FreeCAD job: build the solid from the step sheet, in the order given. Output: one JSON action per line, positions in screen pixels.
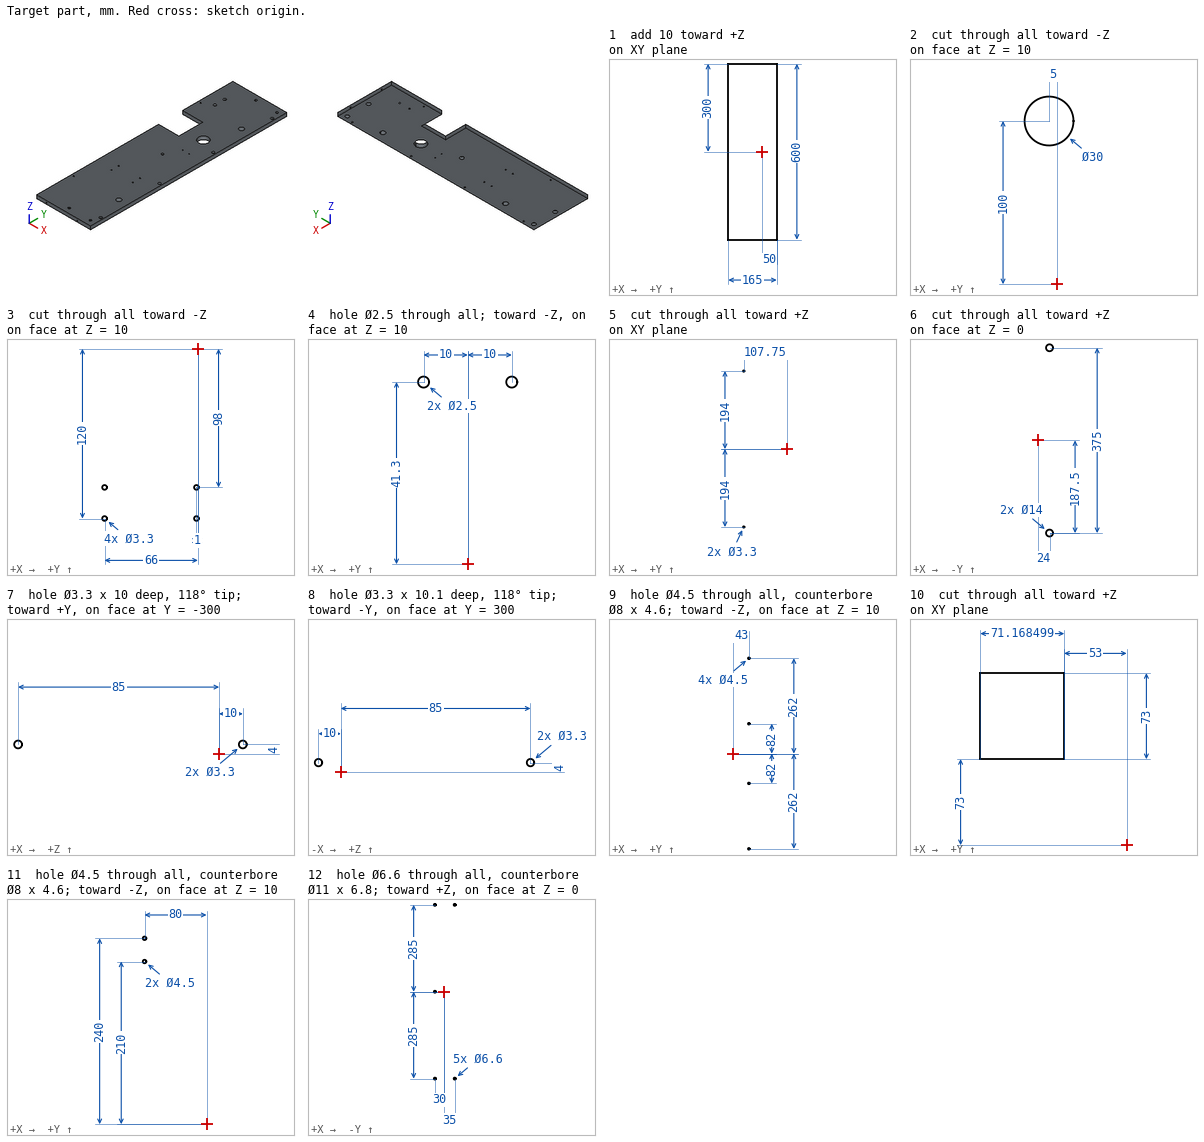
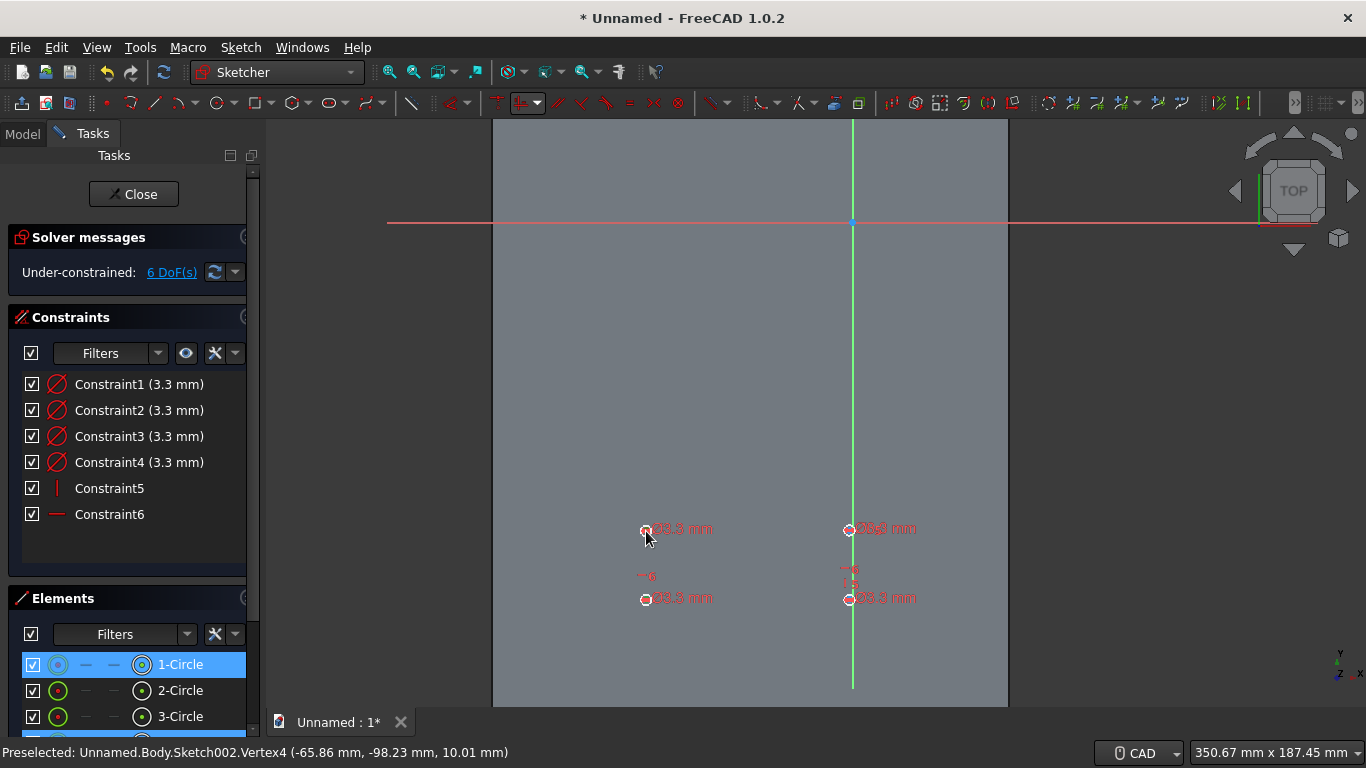
{"action": "left_click", "coordinate": [540, 104]}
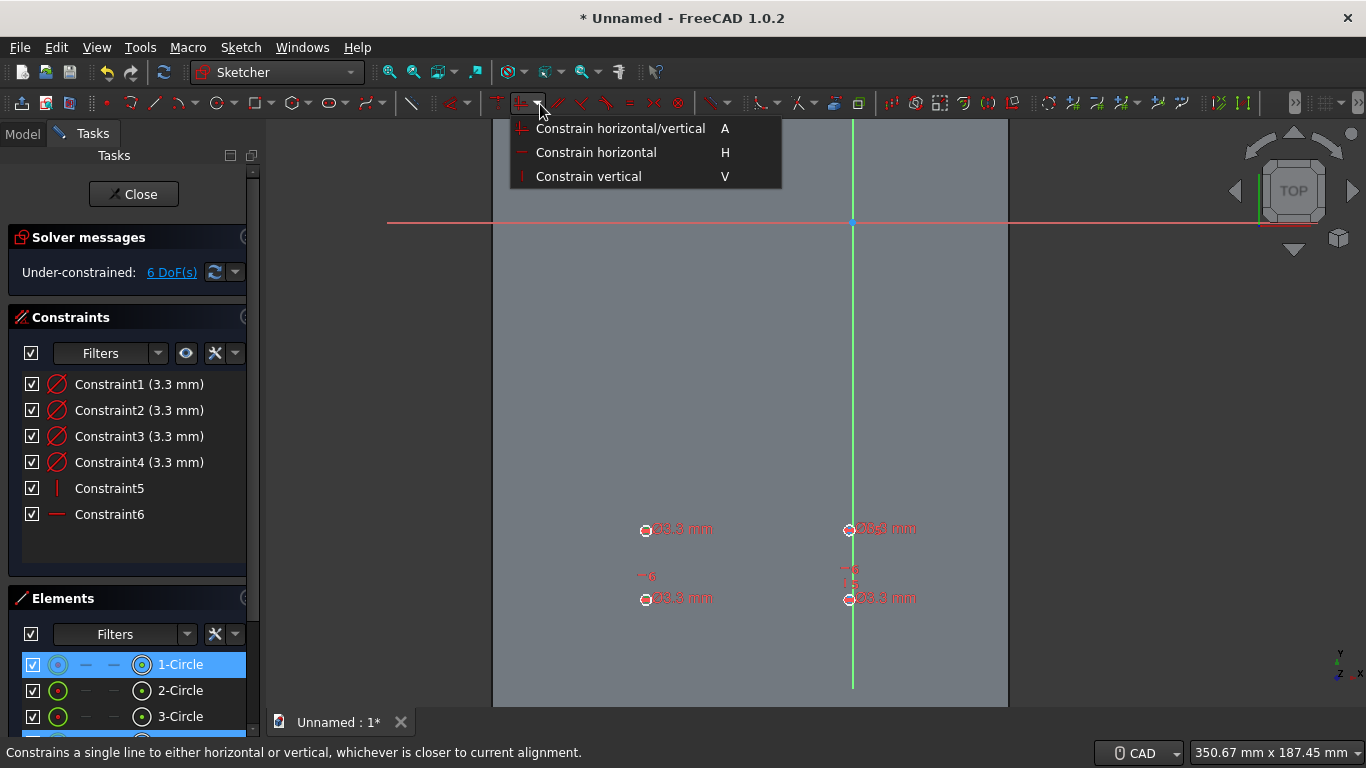
{"action": "left_click", "coordinate": [646, 176]}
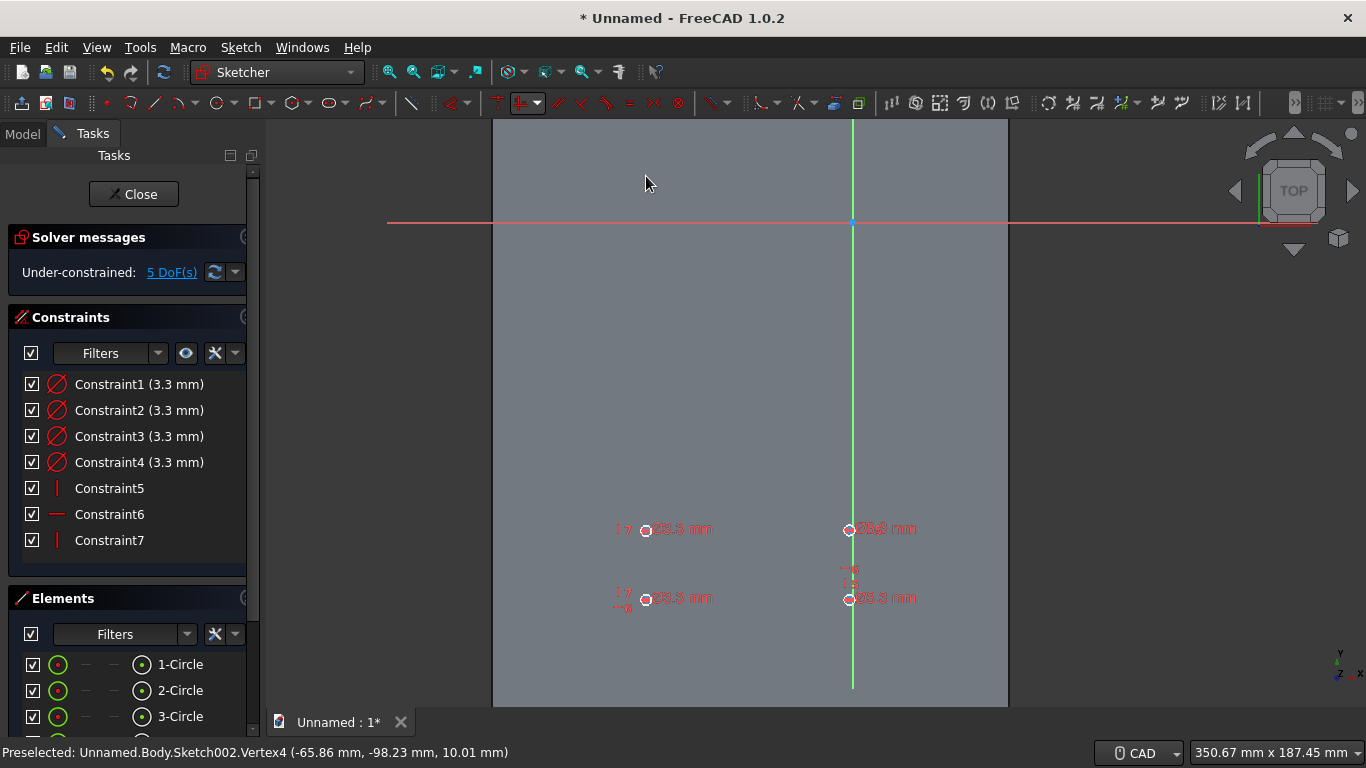
{"action": "left_click", "coordinate": [849, 530]}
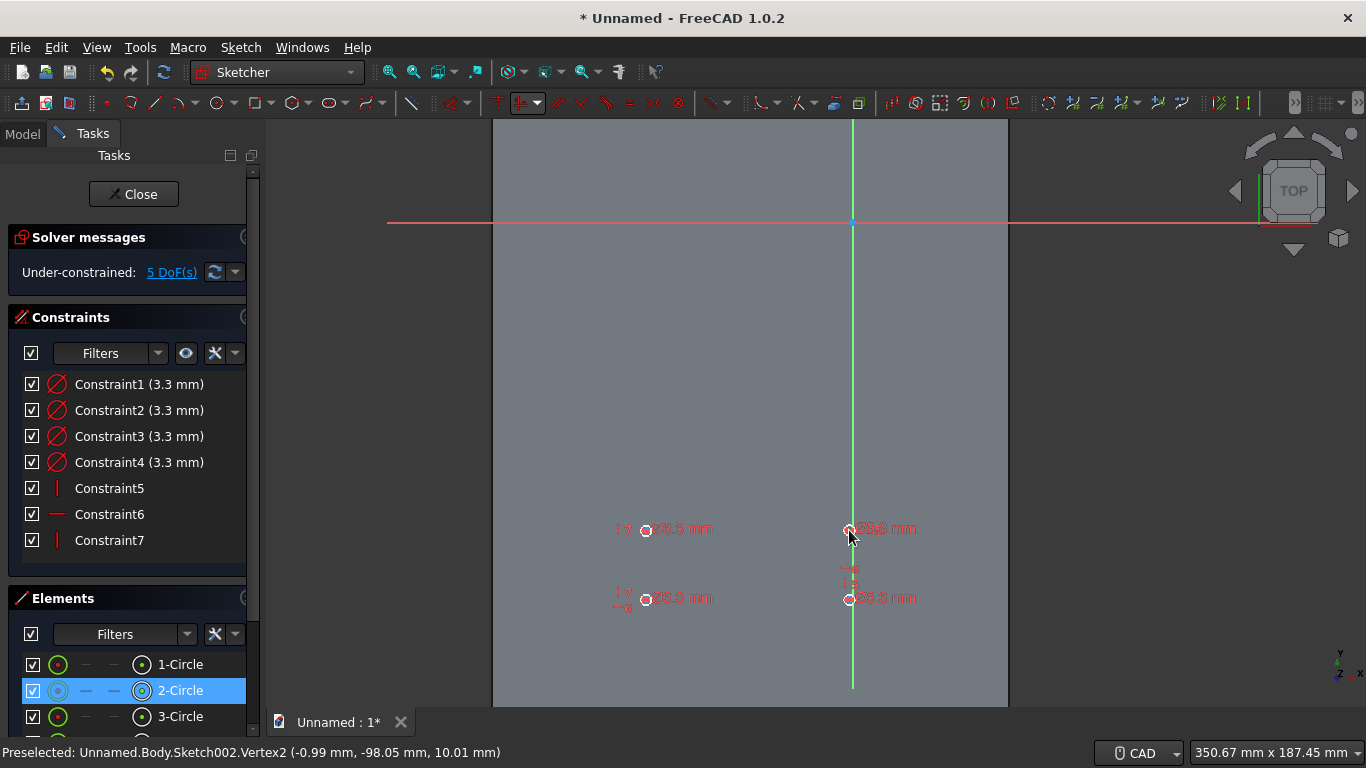
{"action": "left_click", "coordinate": [646, 531]}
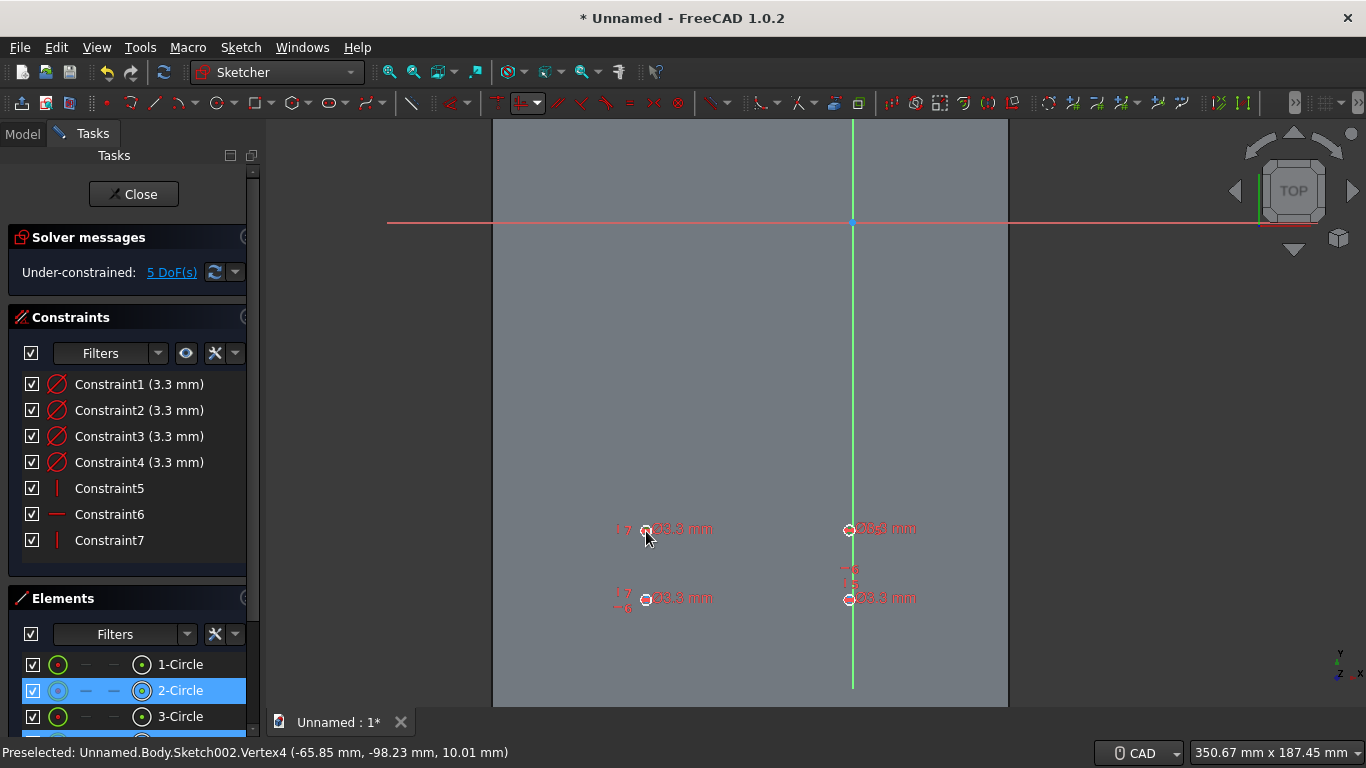
{"action": "left_click", "coordinate": [540, 104]}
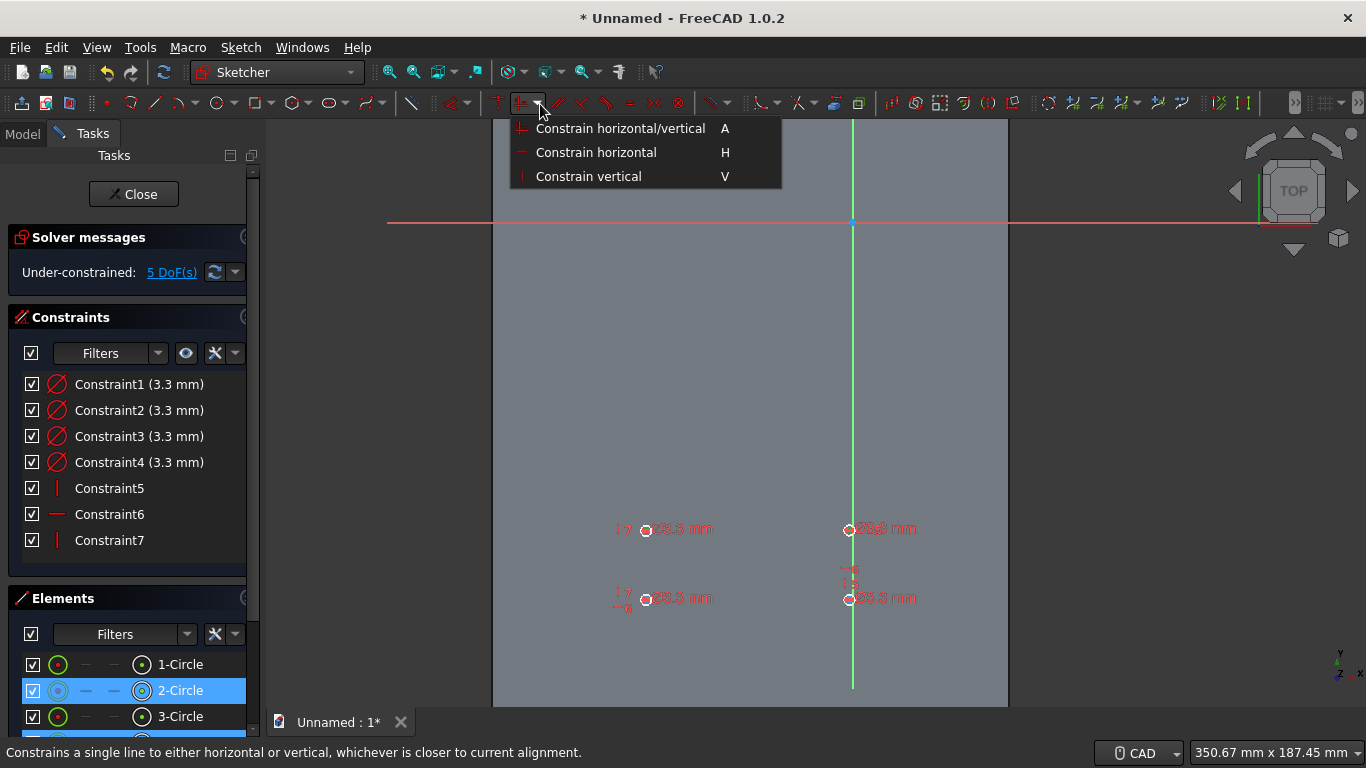
{"action": "left_click", "coordinate": [646, 152]}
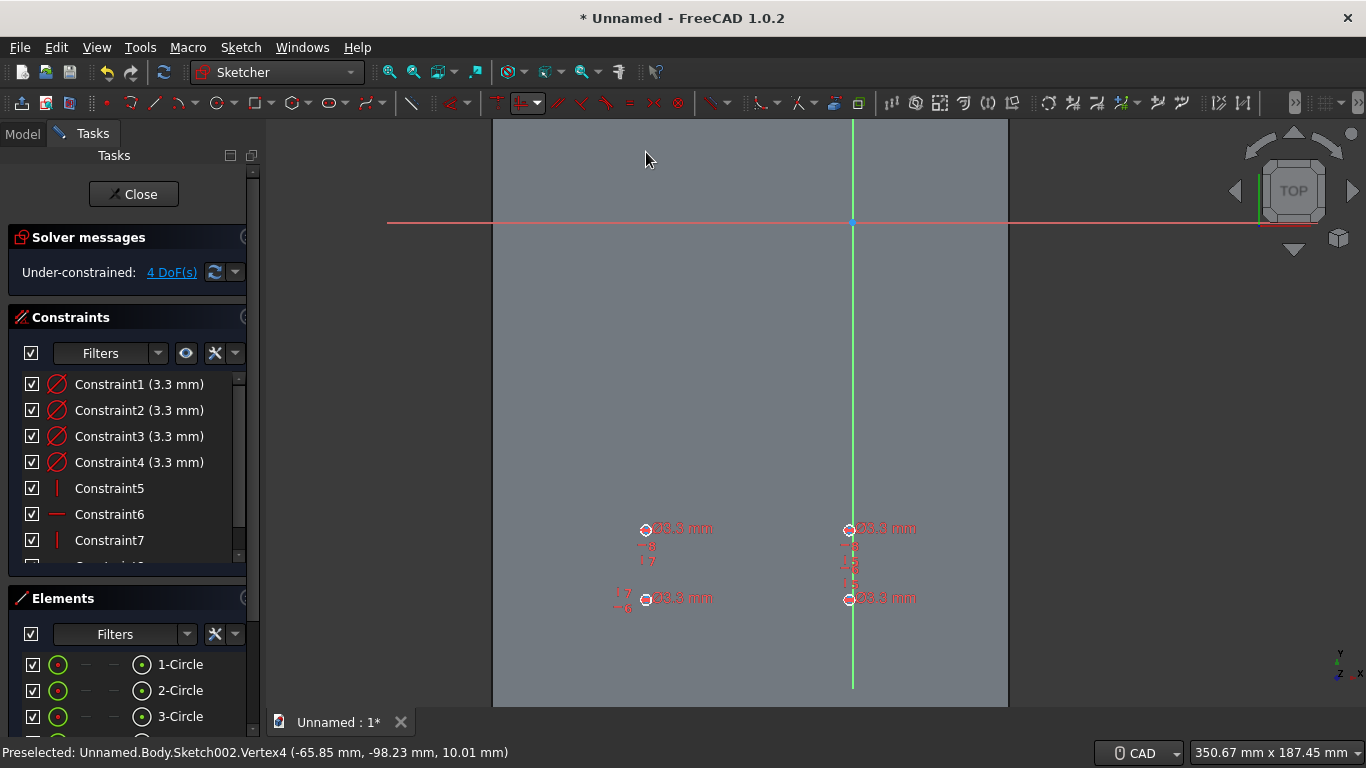
{"action": "left_click", "coordinate": [450, 104]}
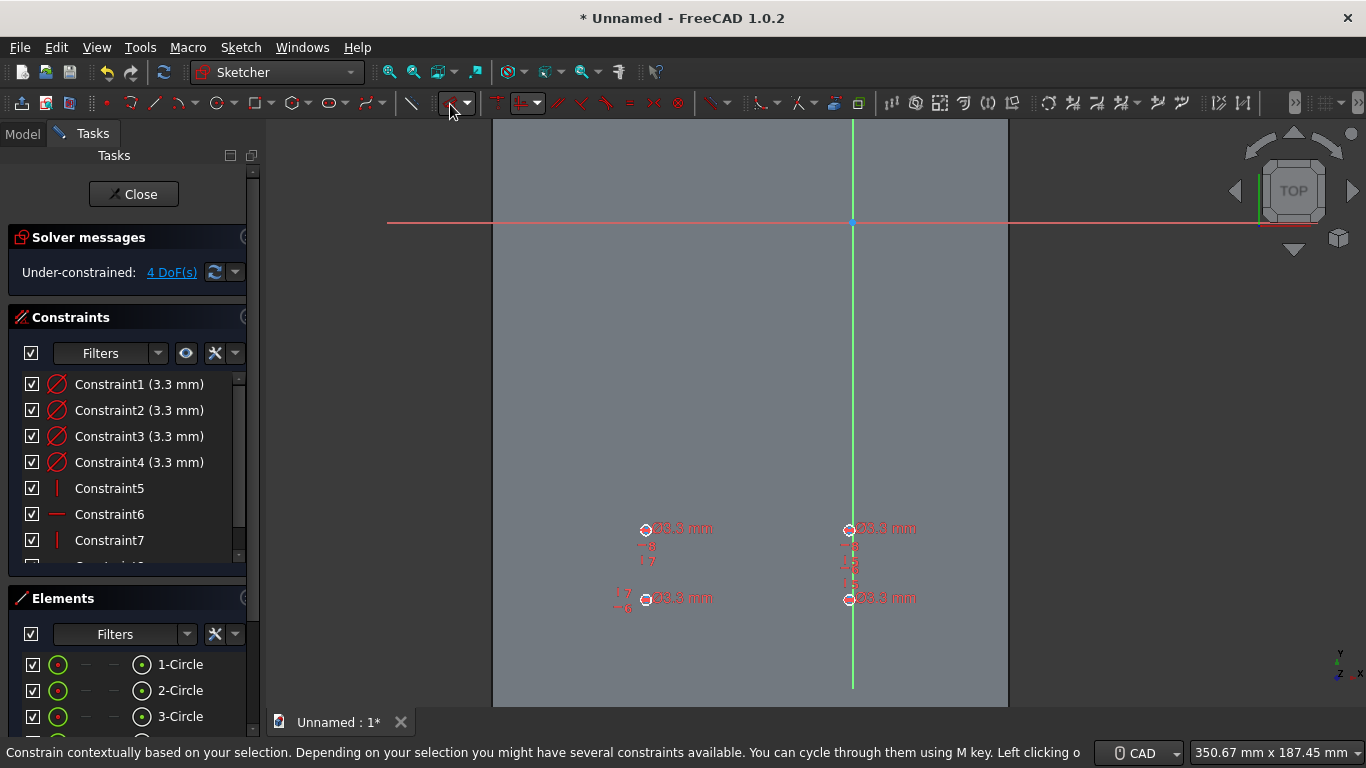
{"action": "scroll", "coordinate": [849, 530], "scroll_direction": "up", "scroll_amount": 13}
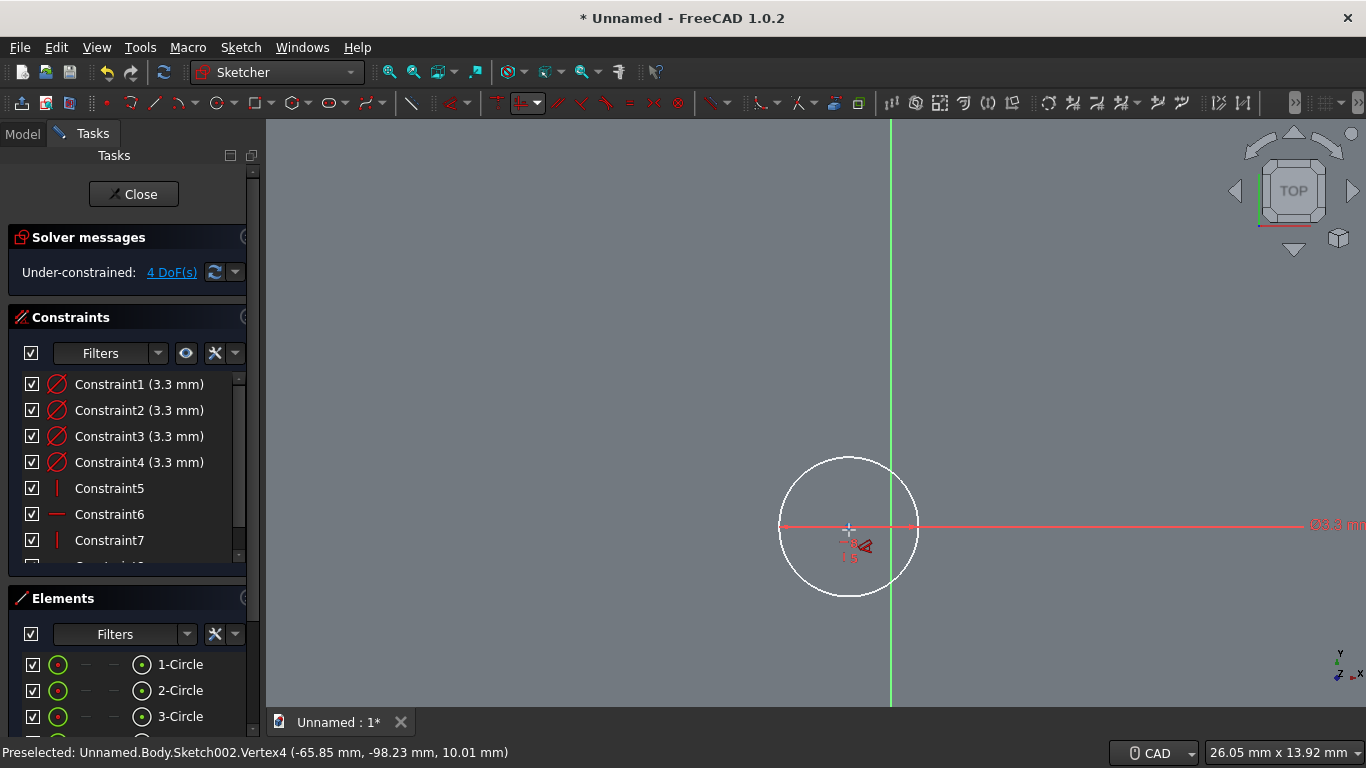
{"action": "left_click", "coordinate": [849, 527]}
{"action": "left_click", "coordinate": [870, 561]}